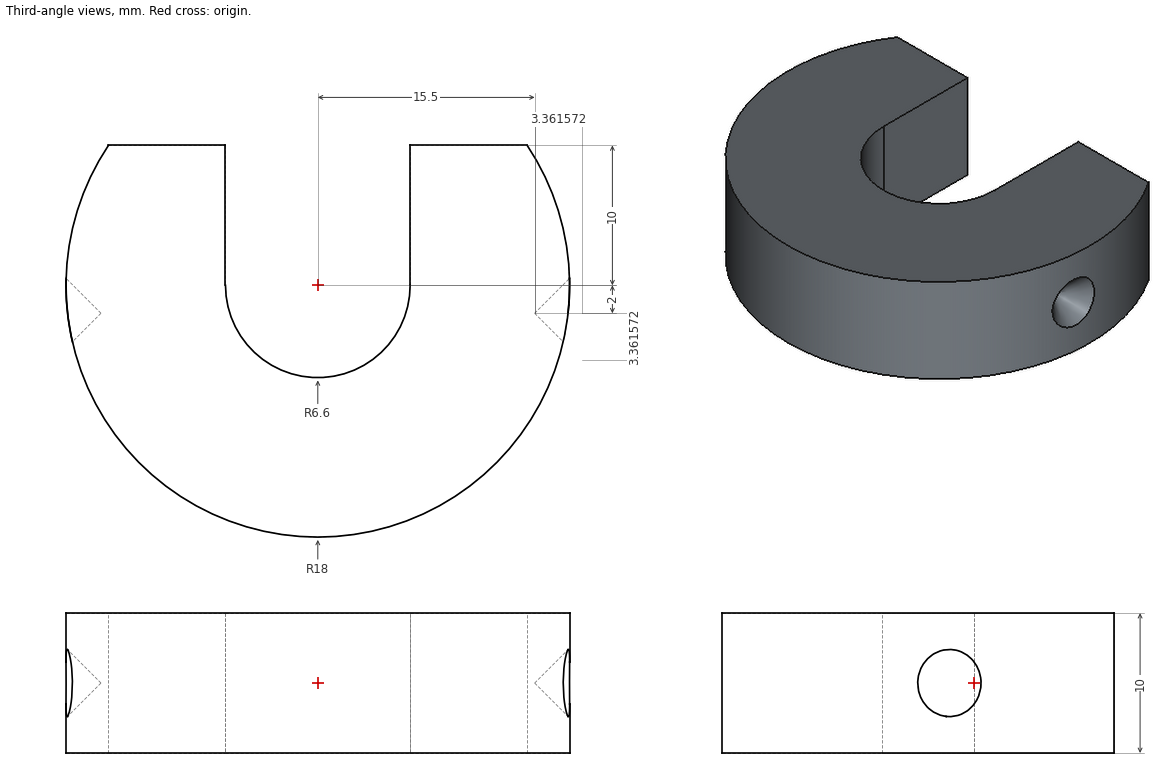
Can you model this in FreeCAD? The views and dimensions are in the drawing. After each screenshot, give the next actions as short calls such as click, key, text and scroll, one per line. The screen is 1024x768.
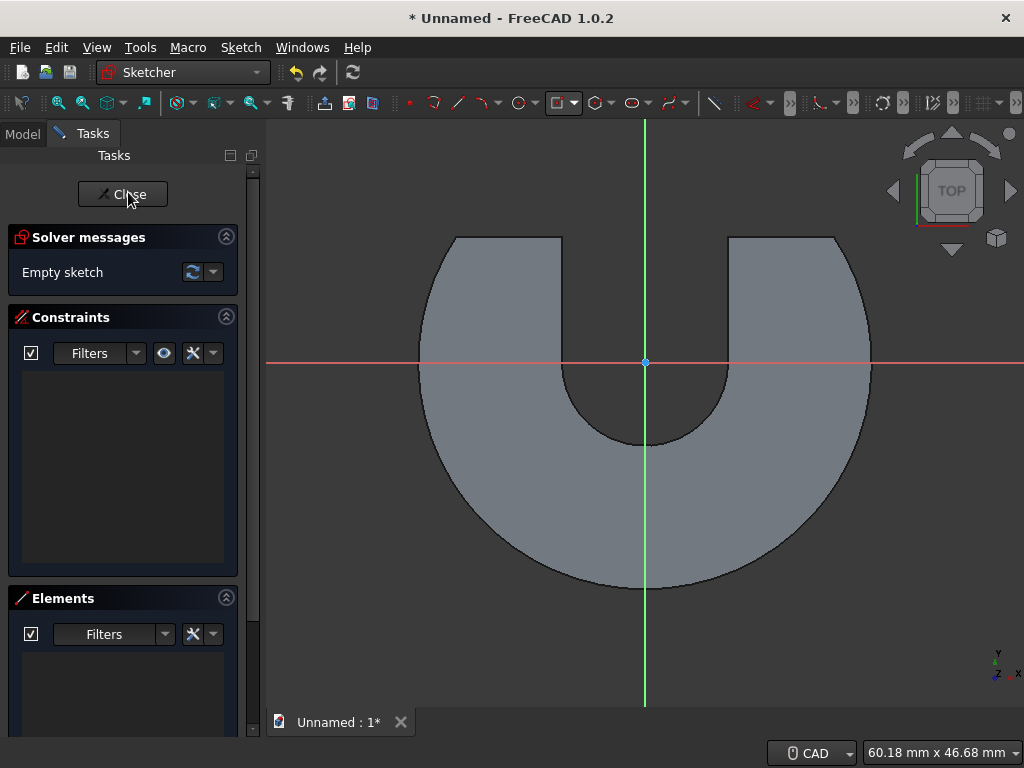
scroll(576, 413, down, 5)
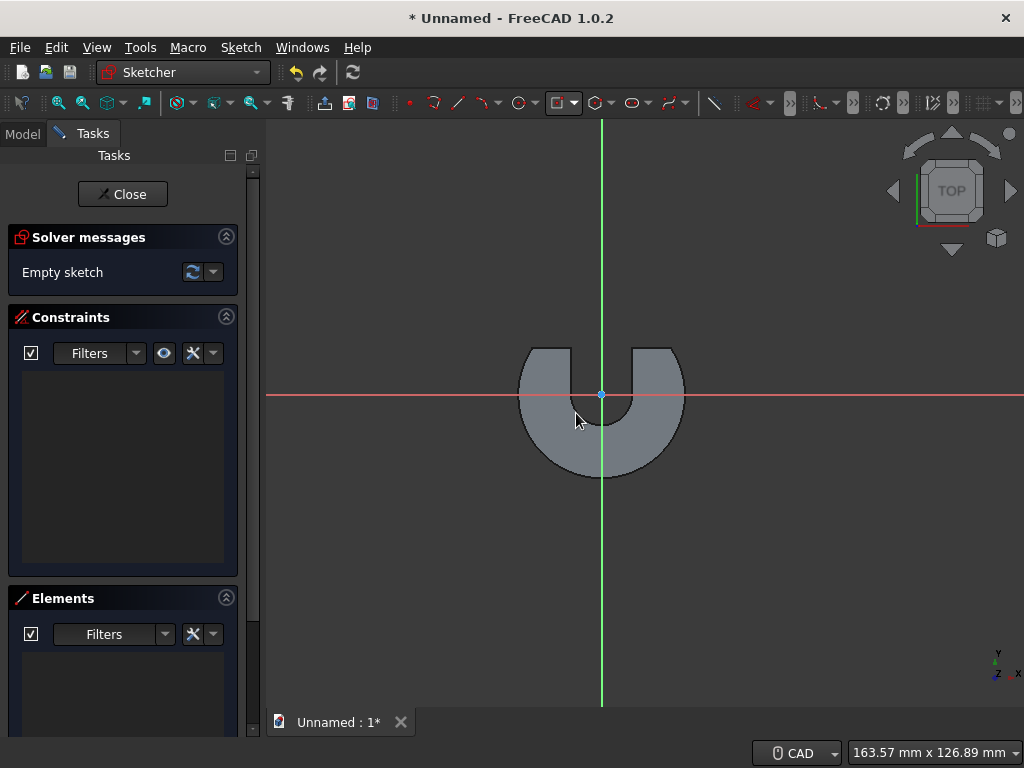
scroll(690, 412, up, 15)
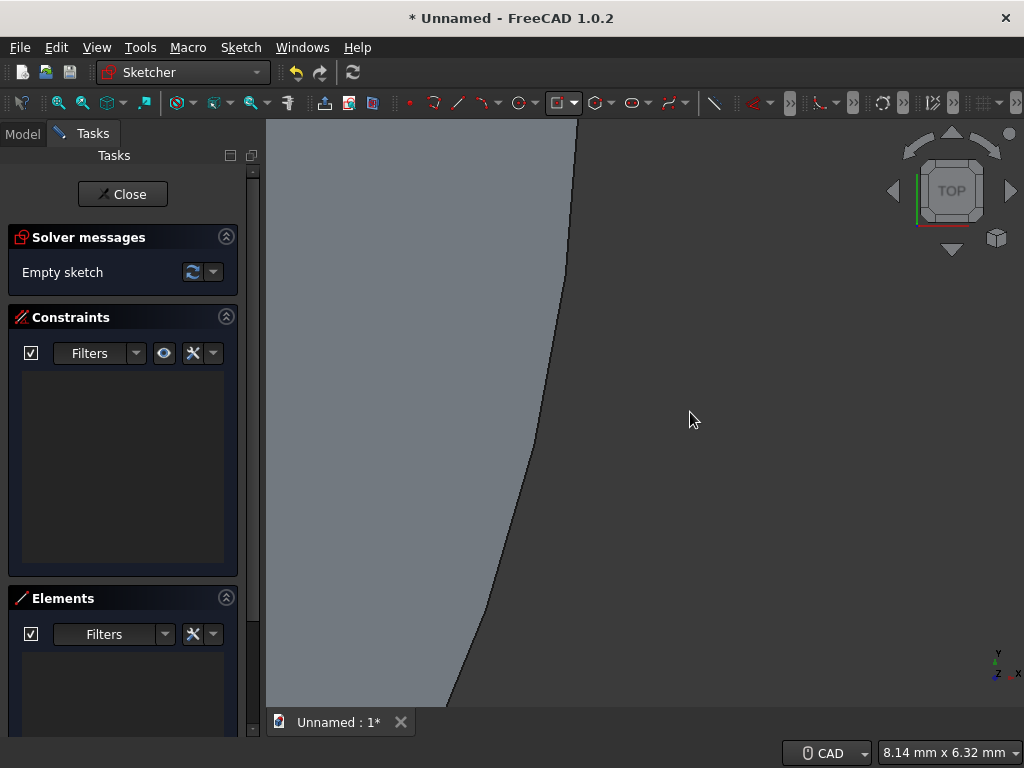
click(434, 104)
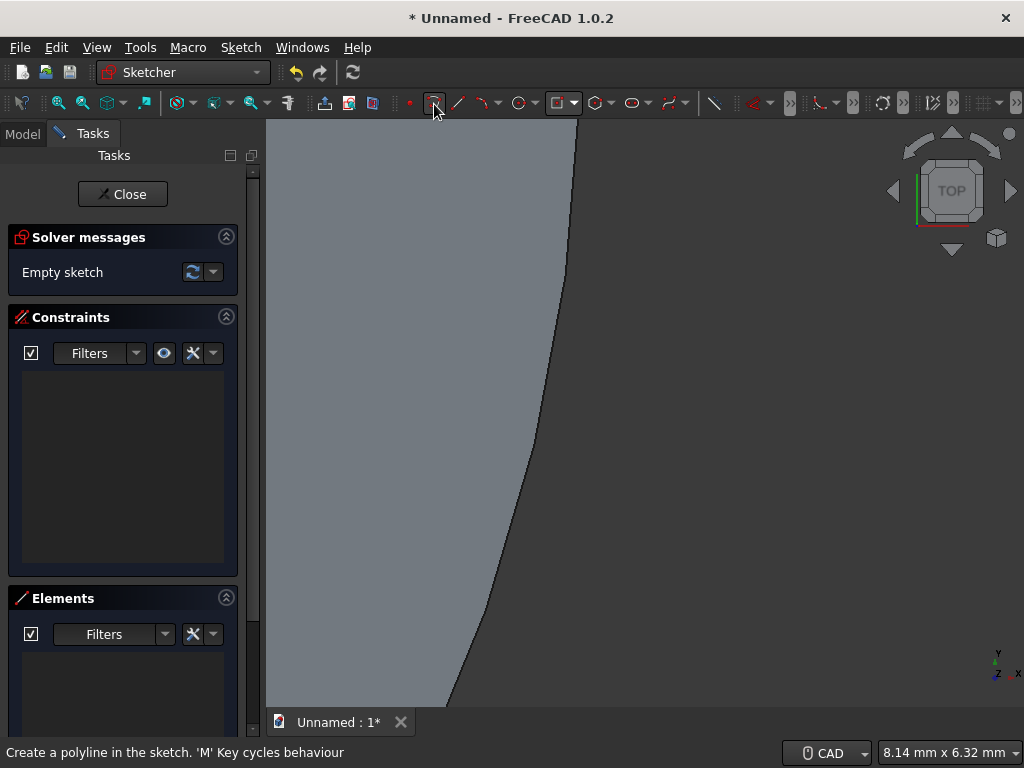
click(347, 243)
click(660, 556)
click(660, 243)
click(347, 244)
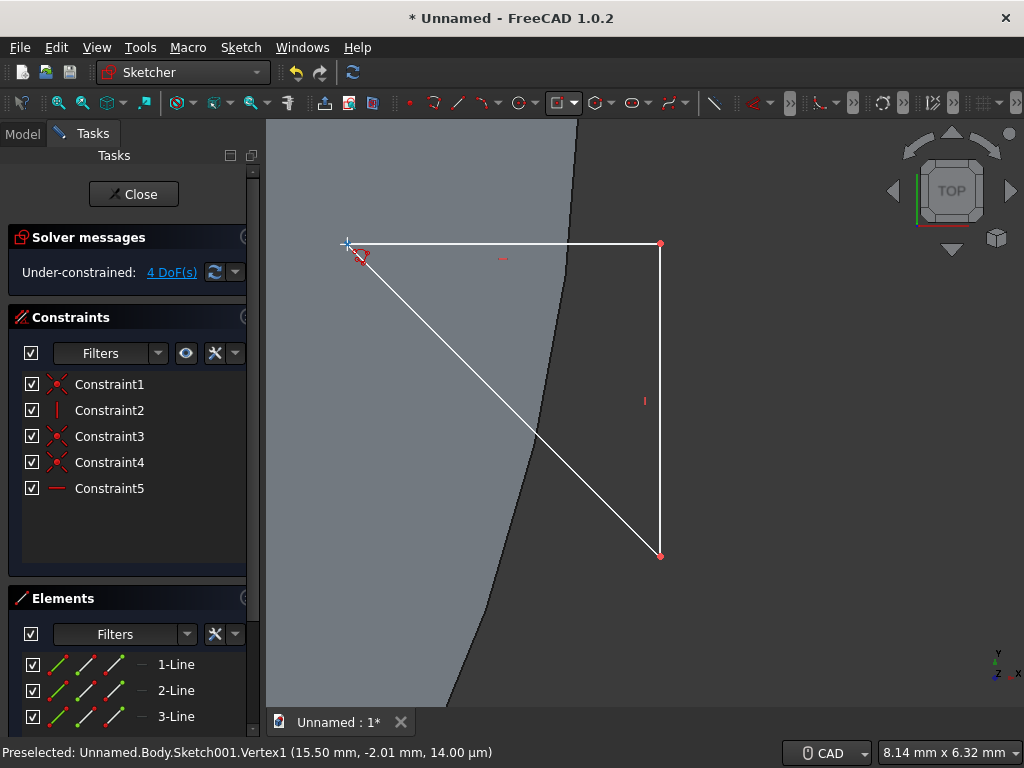
key(g)
key(l)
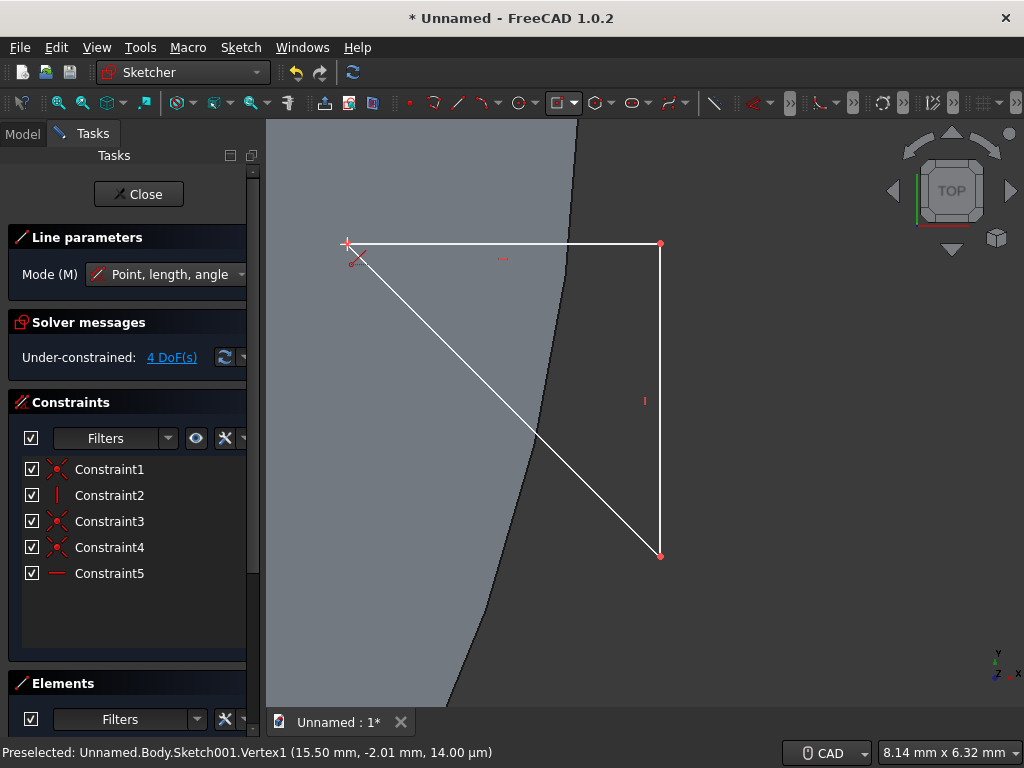
click(691, 243)
click(785, 243)
key(Escape)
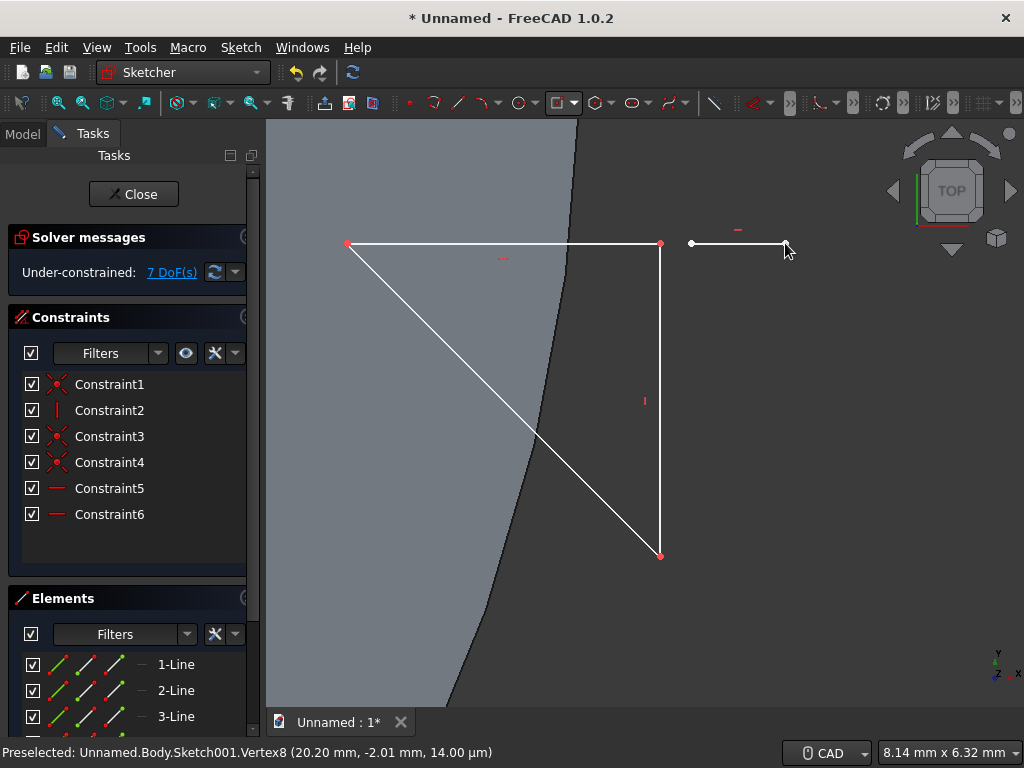
click(719, 244)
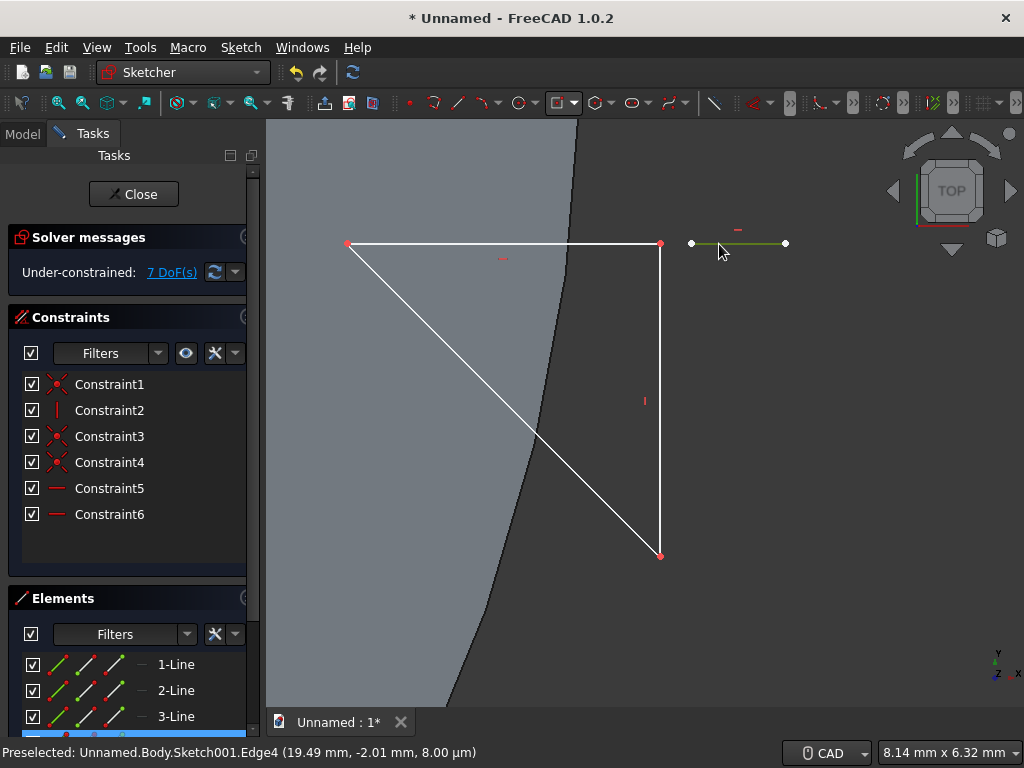
click(716, 104)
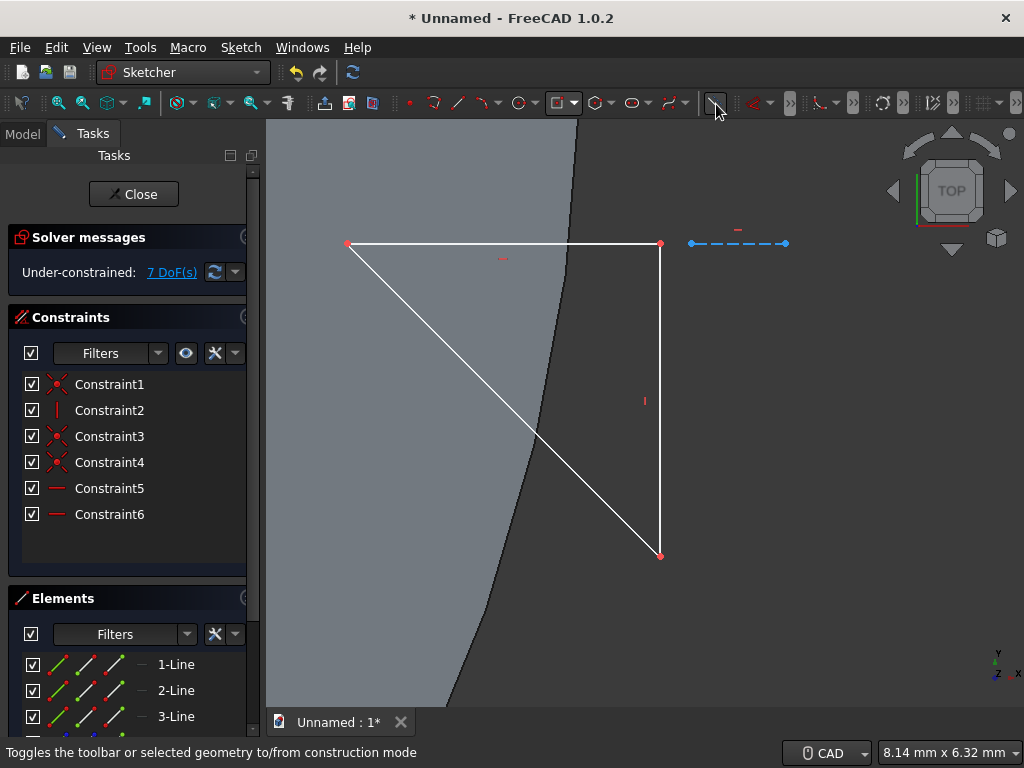
key(d)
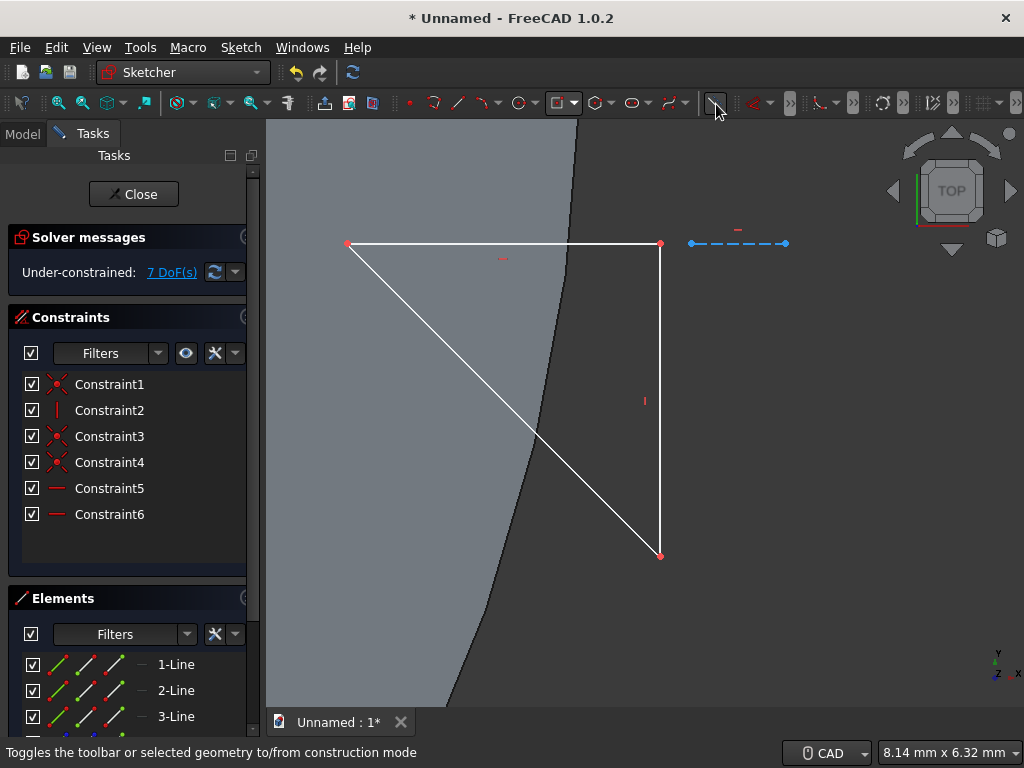
click(347, 244)
click(381, 195)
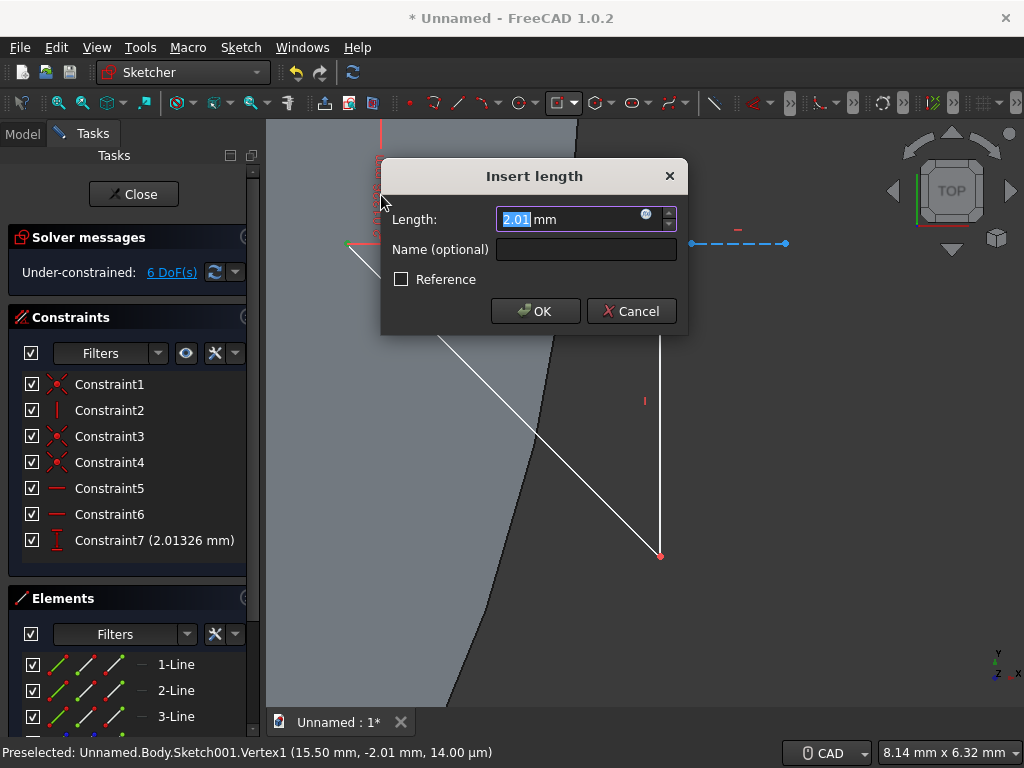
text(2)
key(Return)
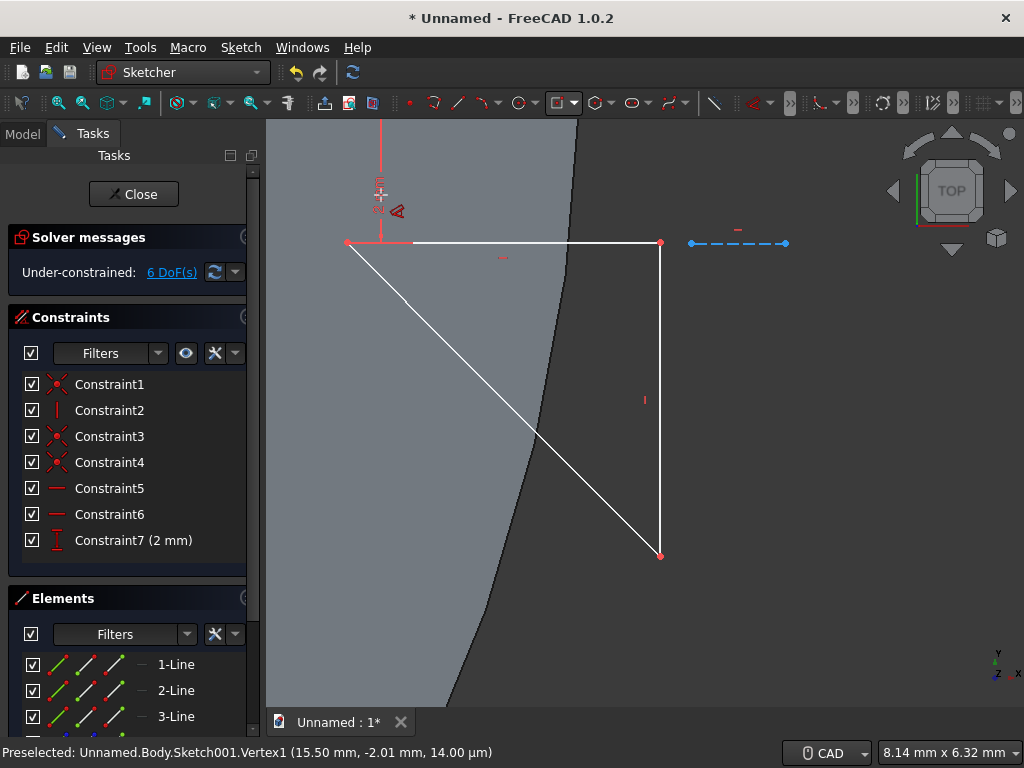
click(691, 244)
click(725, 195)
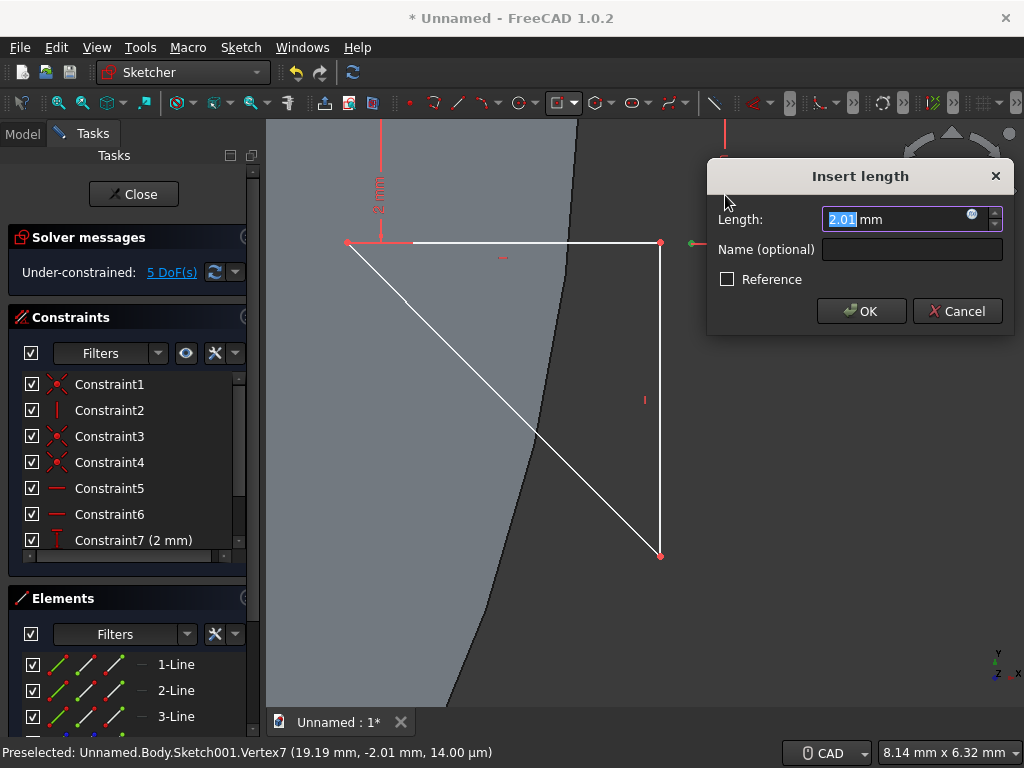
text(2)
key(Return)